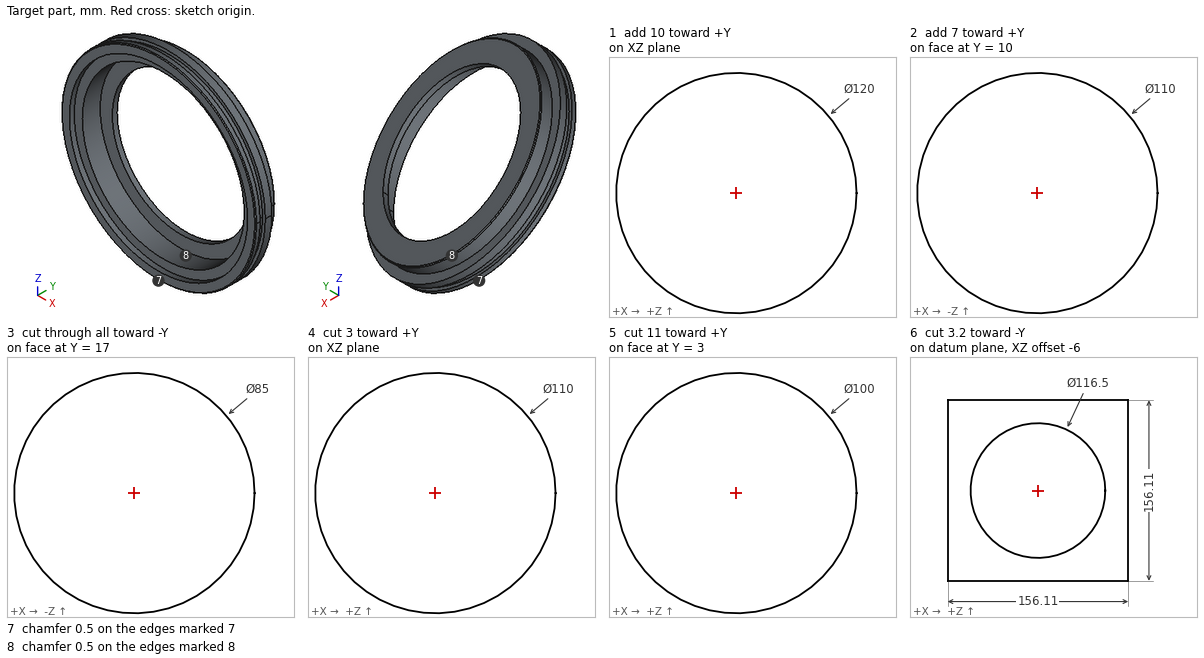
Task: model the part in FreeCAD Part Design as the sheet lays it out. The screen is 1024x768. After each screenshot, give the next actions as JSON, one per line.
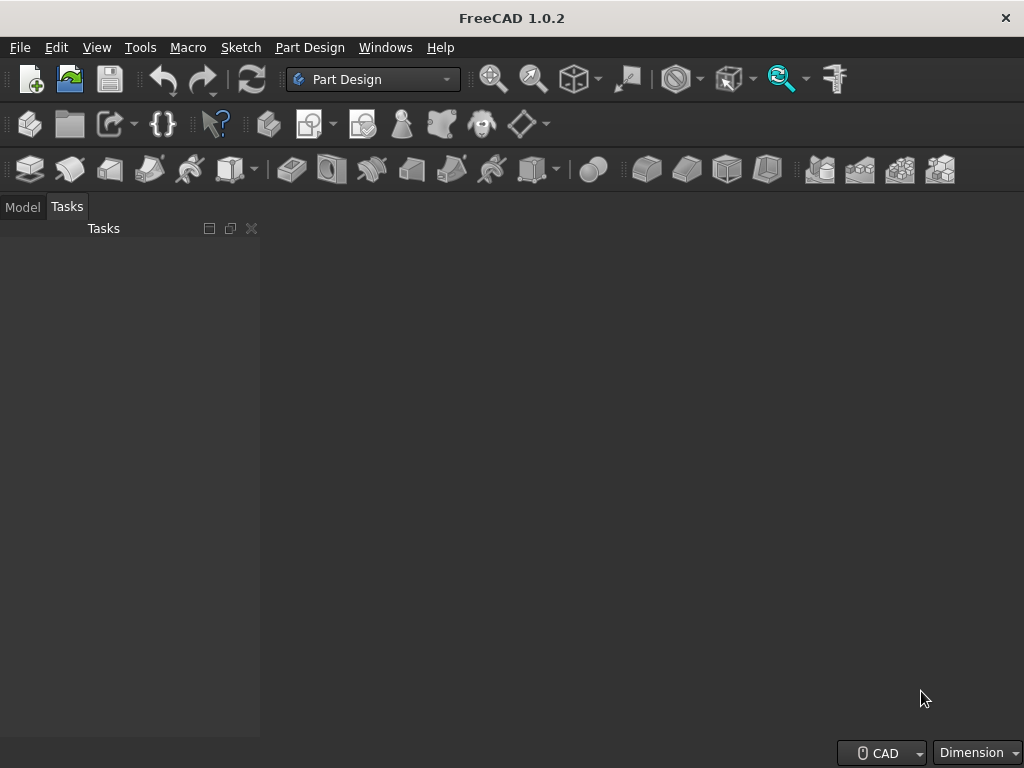
{"action": "key", "text": "ctrl+n"}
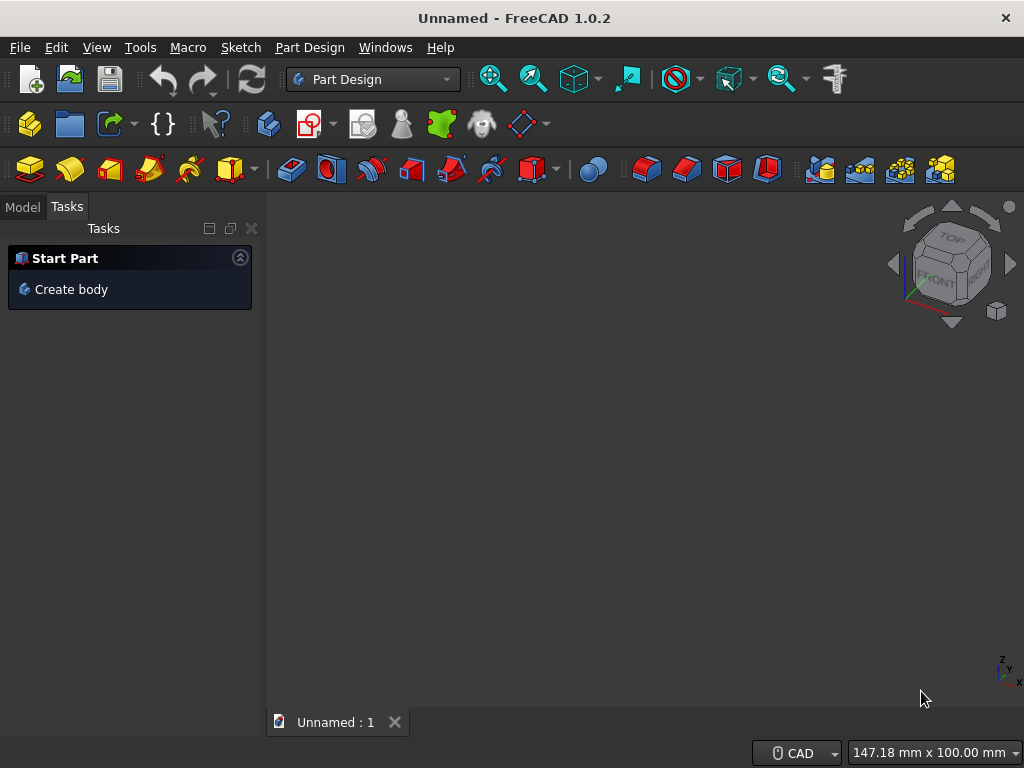
{"action": "left_click", "coordinate": [310, 124]}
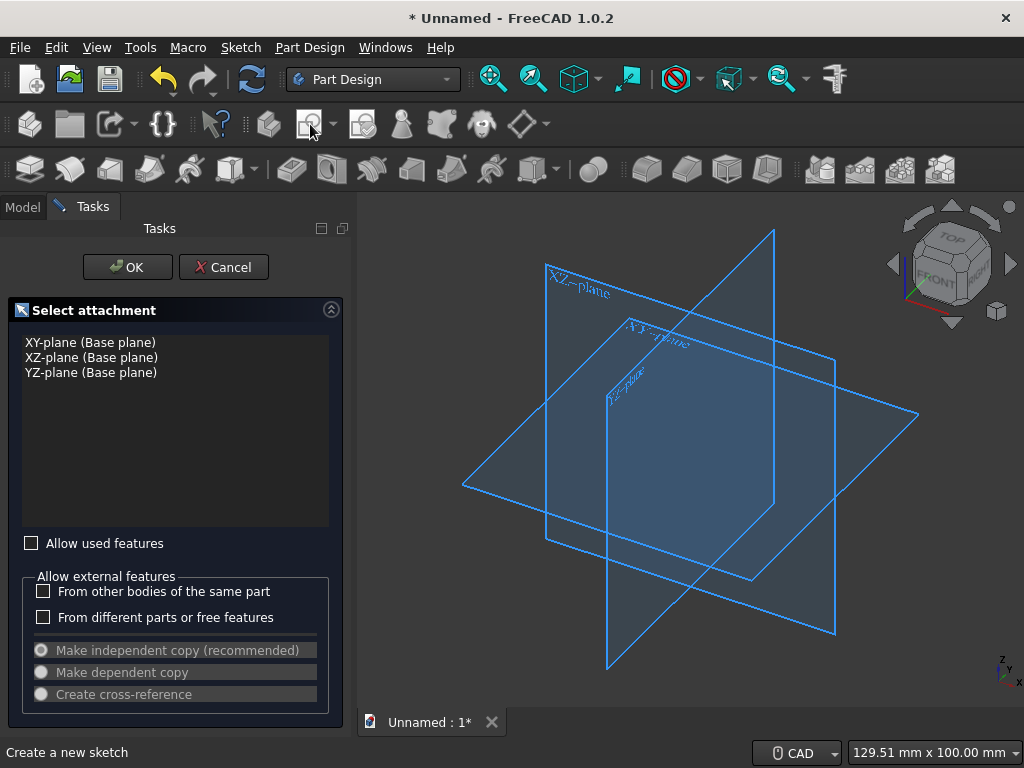
{"action": "left_click", "coordinate": [82, 358]}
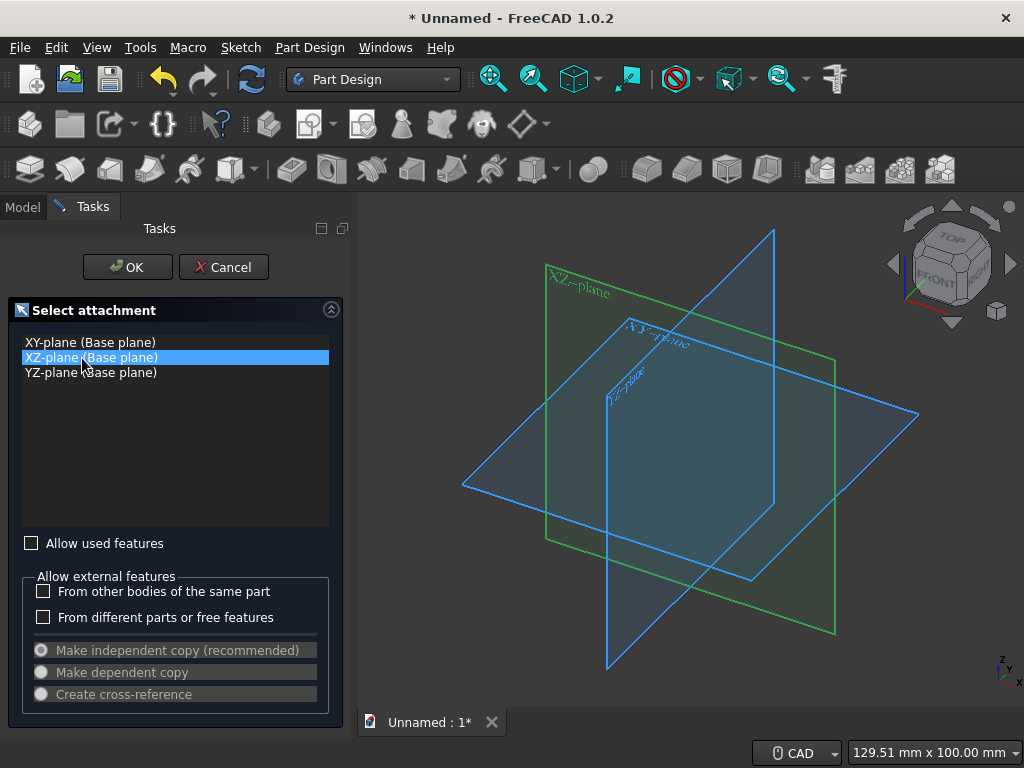
{"action": "left_click", "coordinate": [128, 267]}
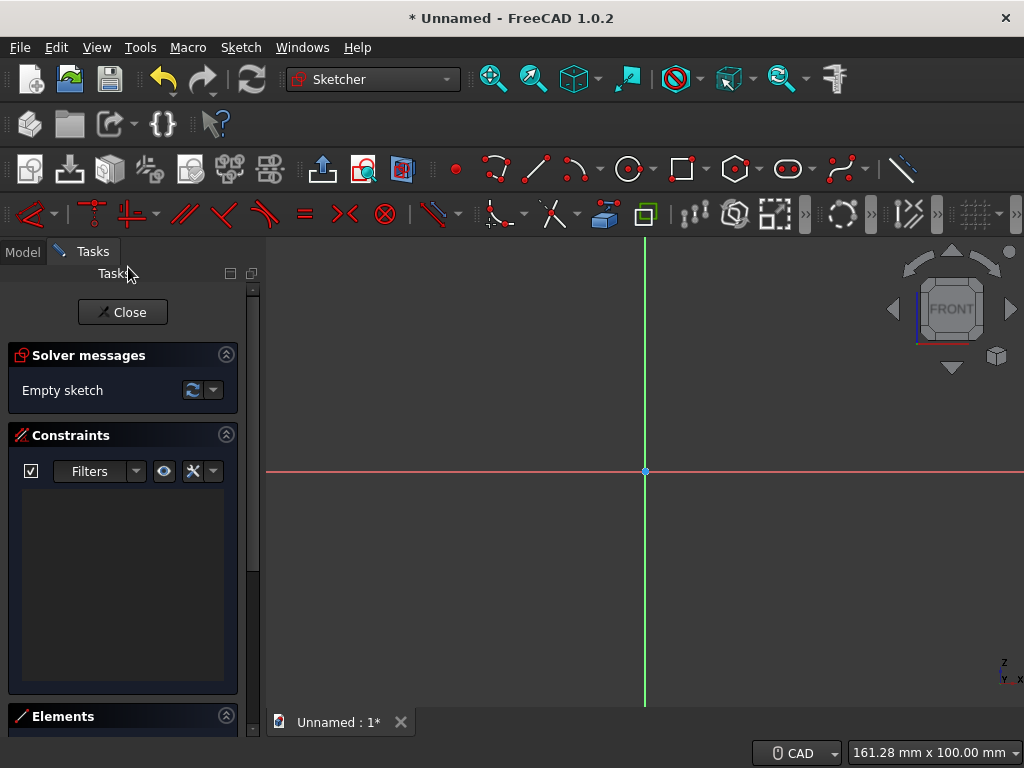
{"action": "scroll", "coordinate": [493, 472], "scroll_direction": "down", "scroll_amount": 3}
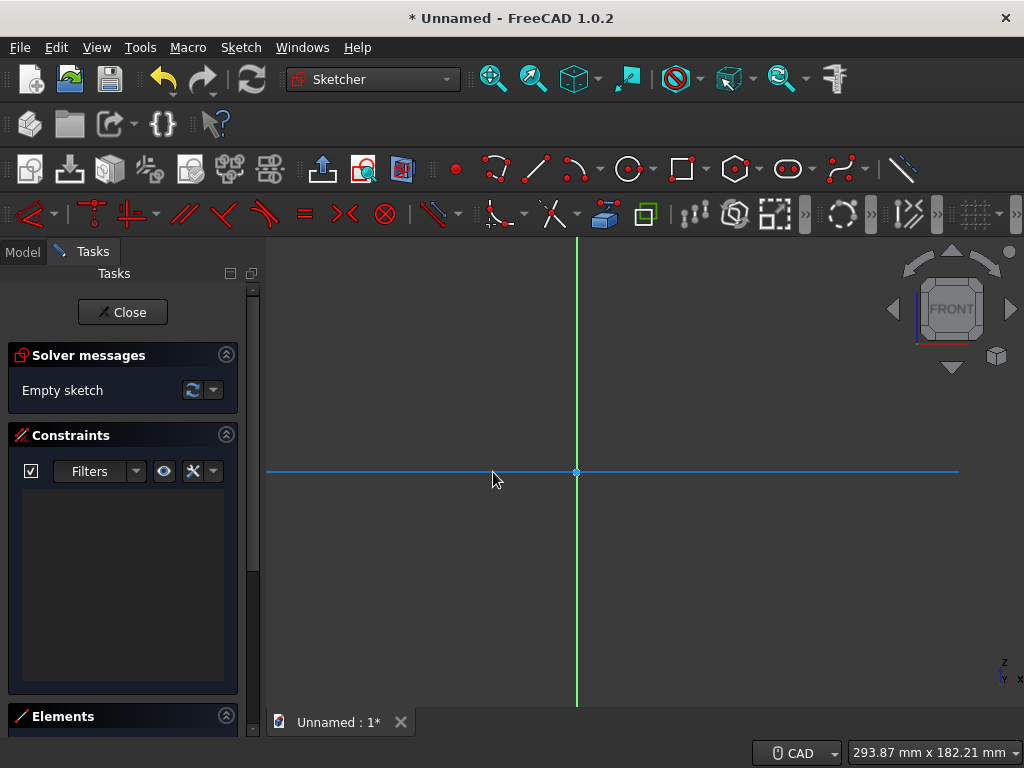
{"action": "left_click", "coordinate": [630, 170]}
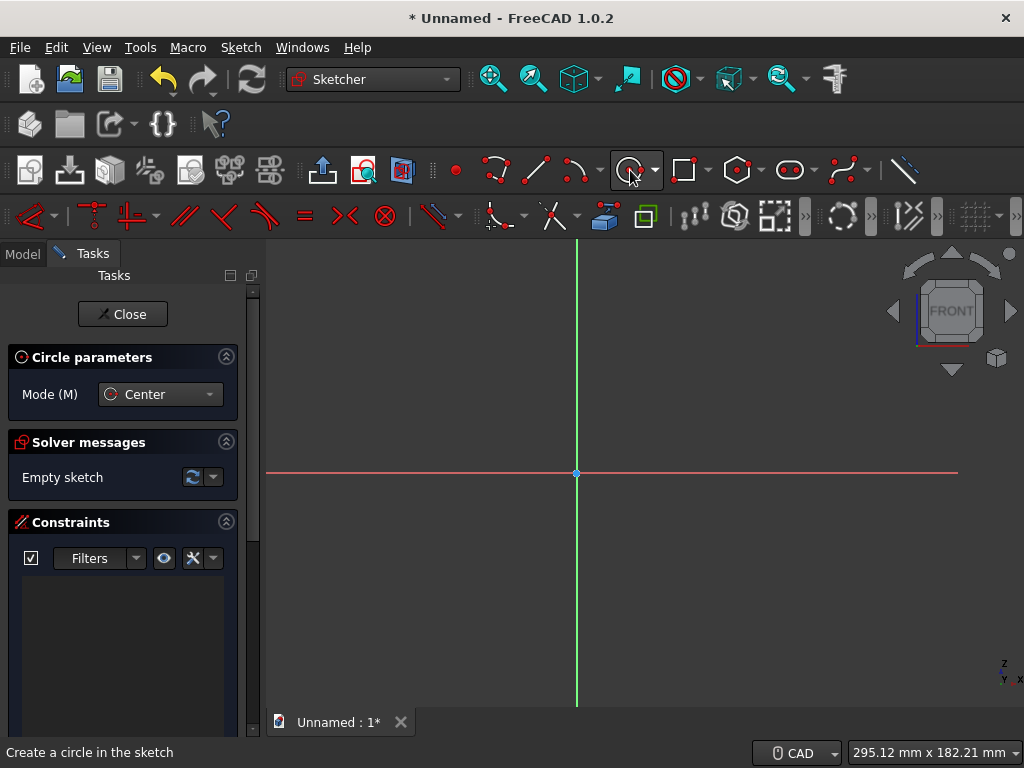
{"action": "left_click", "coordinate": [577, 473]}
{"action": "mouse_move", "coordinate": [686, 364]}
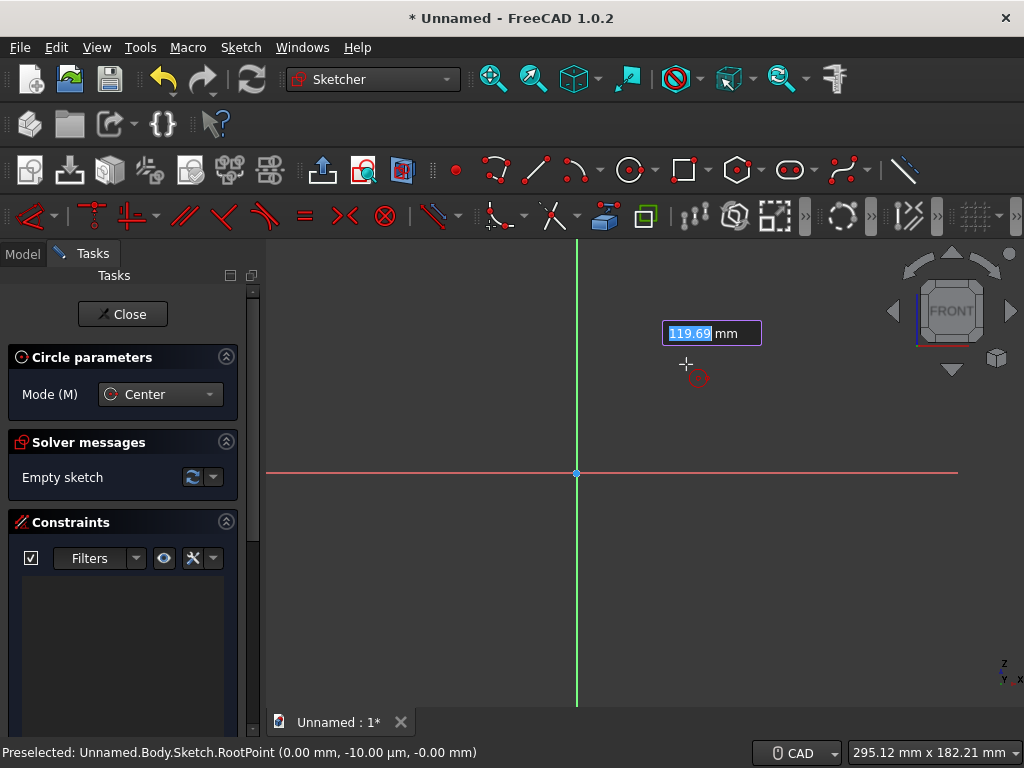
{"action": "type", "text": "120"}
{"action": "key", "text": "Return"}
{"action": "key", "text": "Escape"}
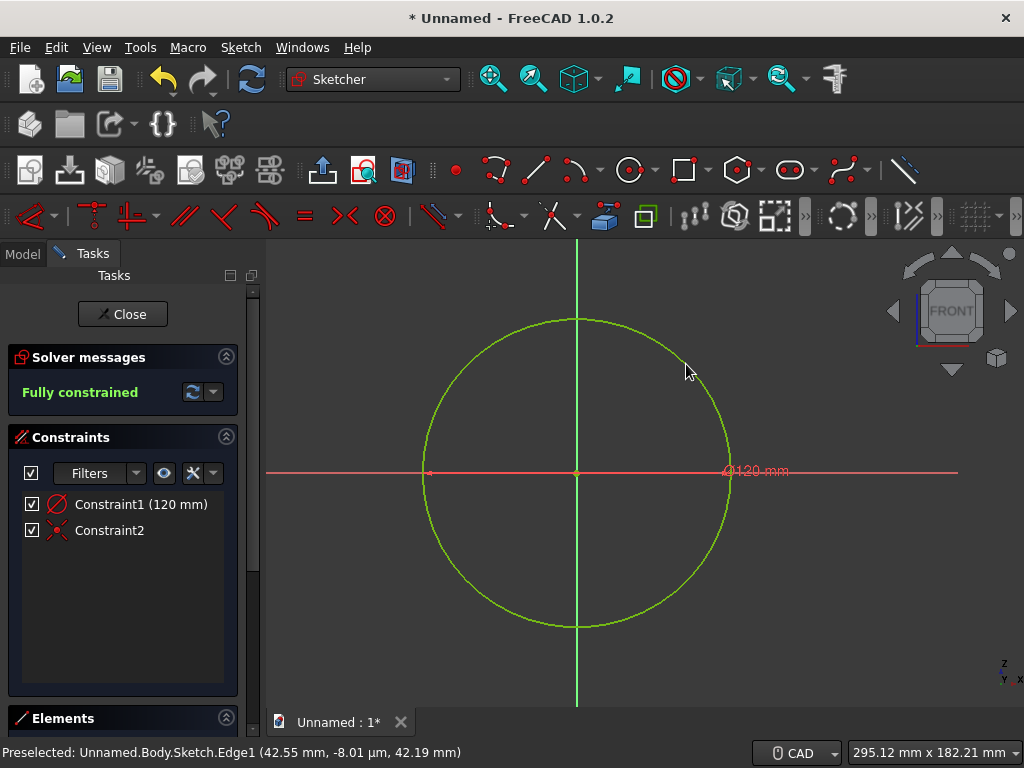
{"action": "left_click", "coordinate": [123, 314]}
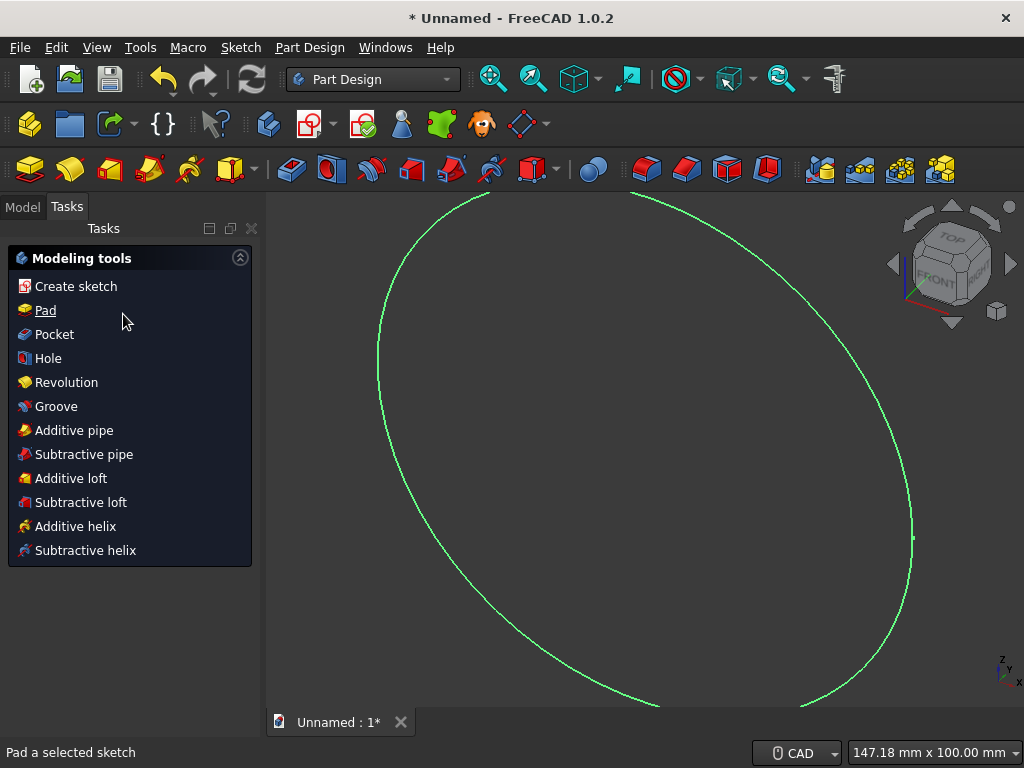
{"action": "left_click", "coordinate": [30, 170]}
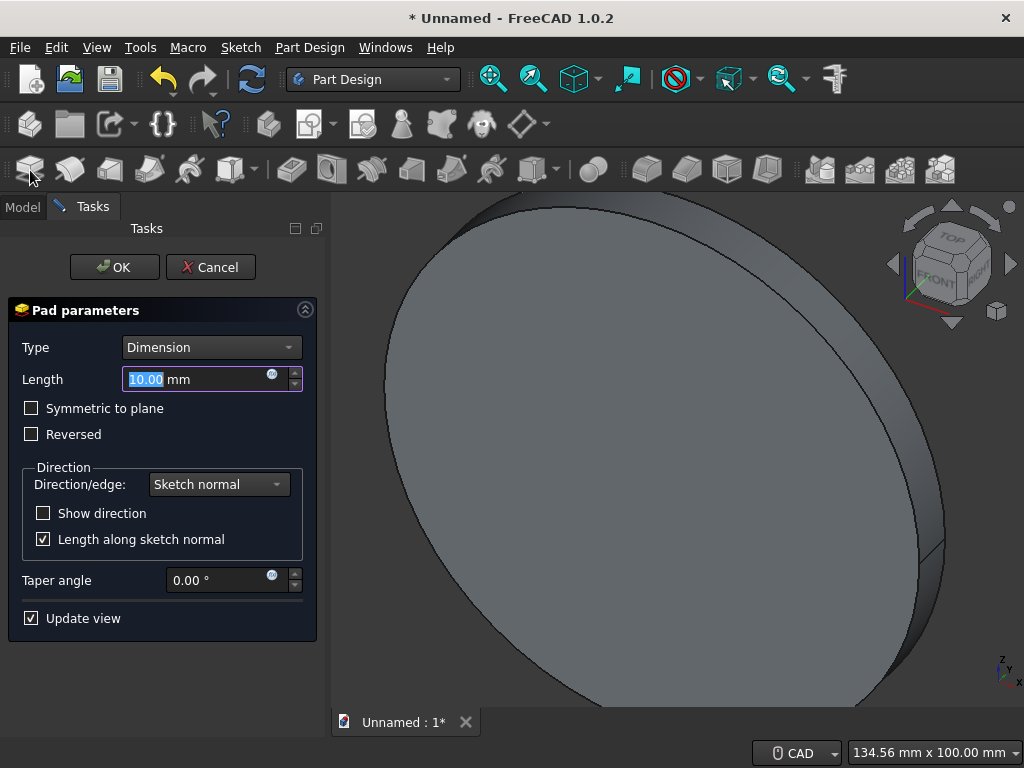
{"action": "type", "text": "10"}
{"action": "key", "text": "Tab"}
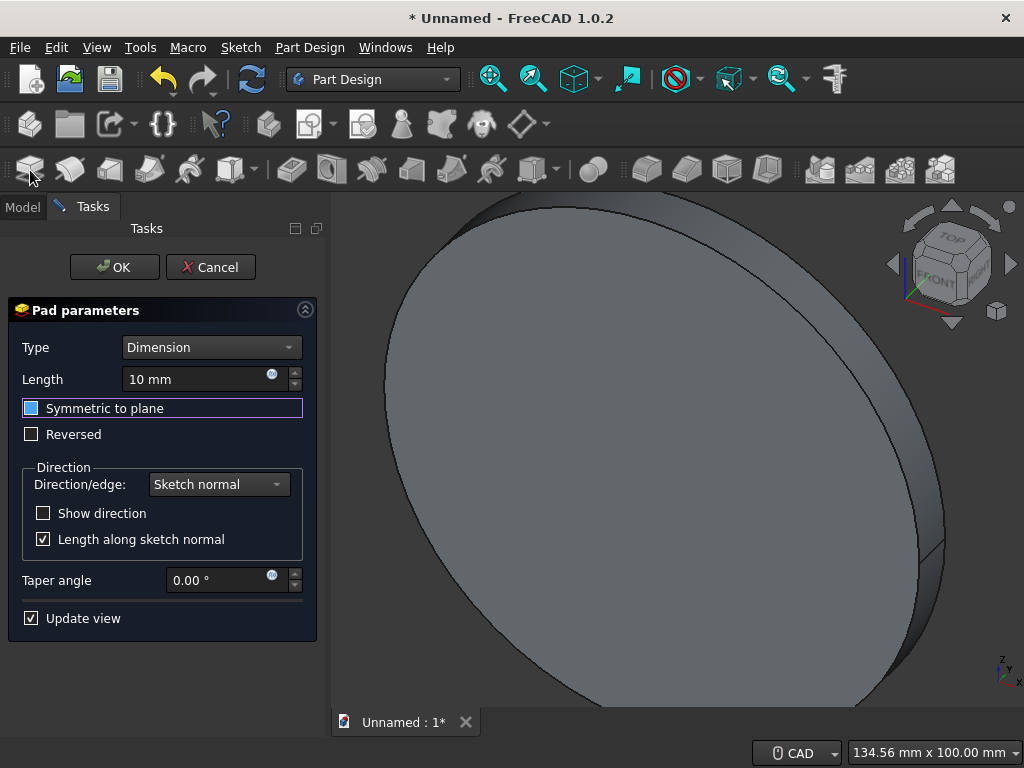
{"action": "left_click", "coordinate": [30, 434]}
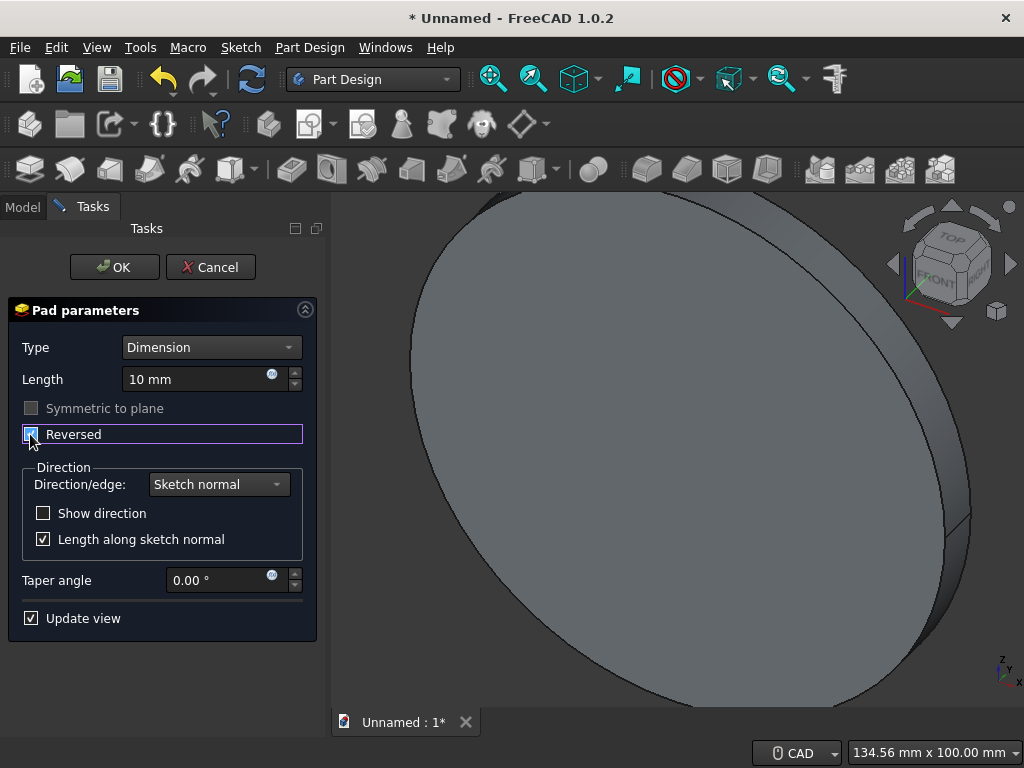
{"action": "left_click", "coordinate": [115, 267]}